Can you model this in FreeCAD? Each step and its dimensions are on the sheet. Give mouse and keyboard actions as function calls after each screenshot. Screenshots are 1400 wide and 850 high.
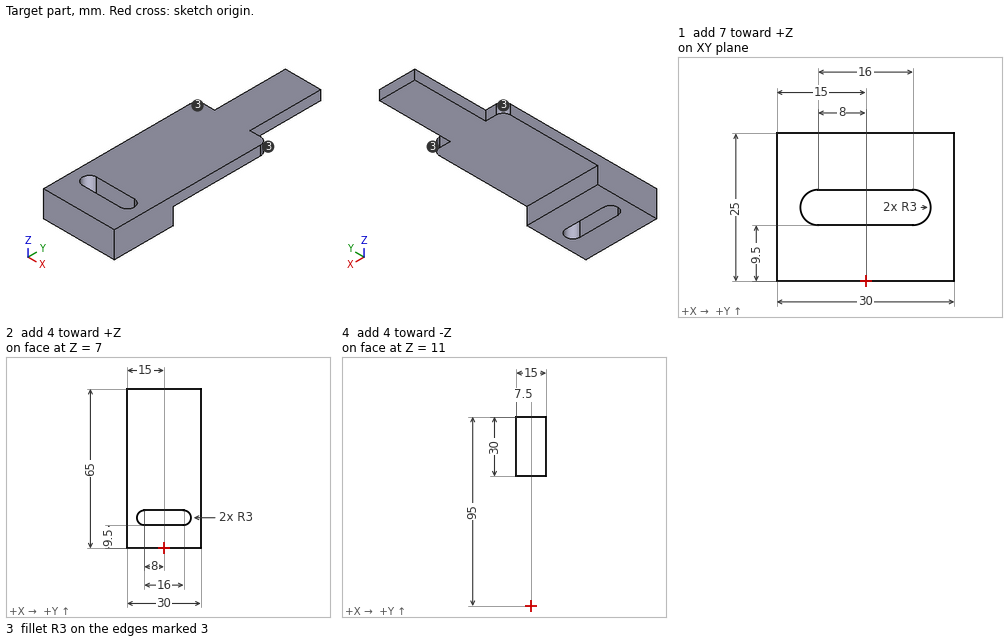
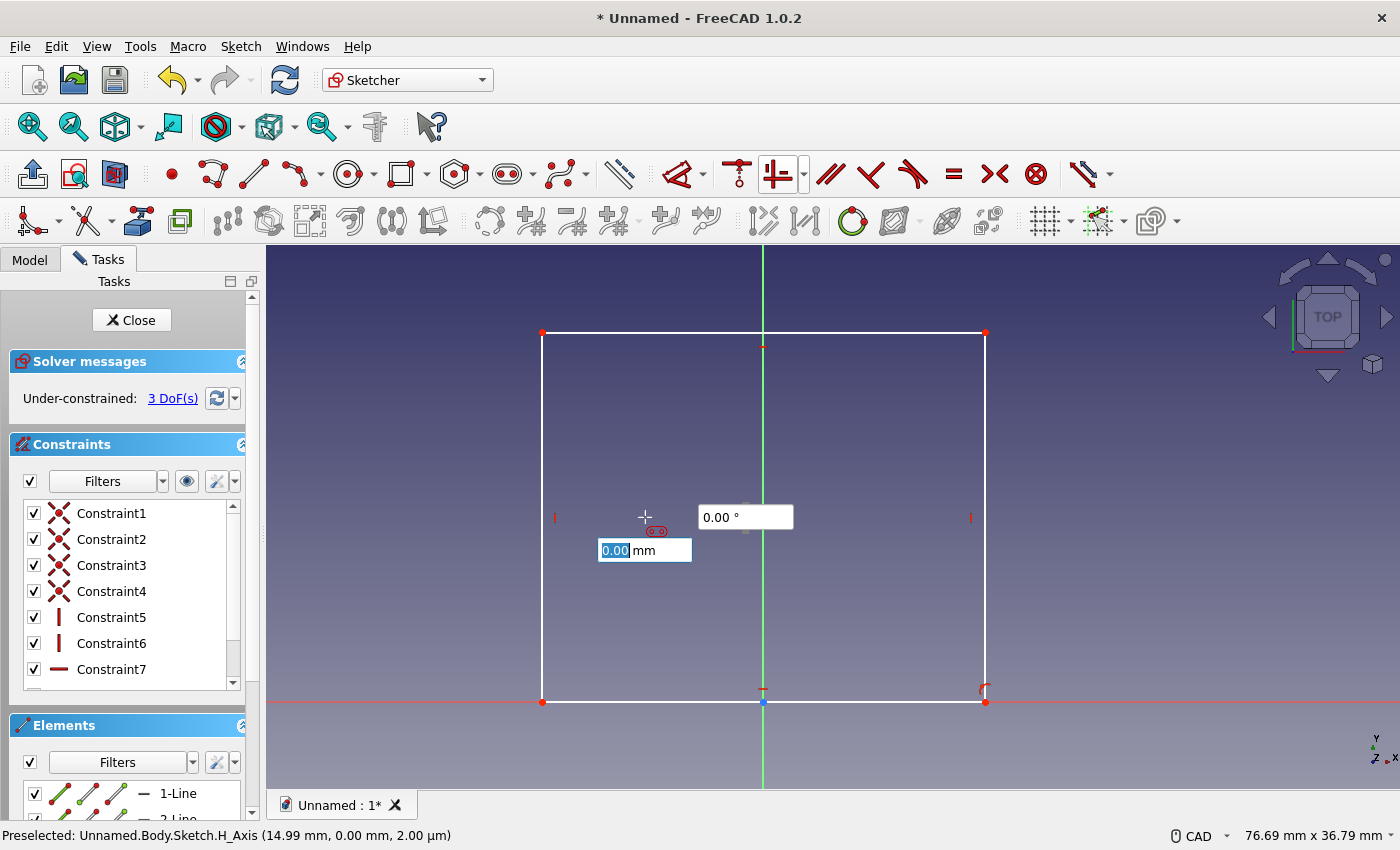
click(882, 517)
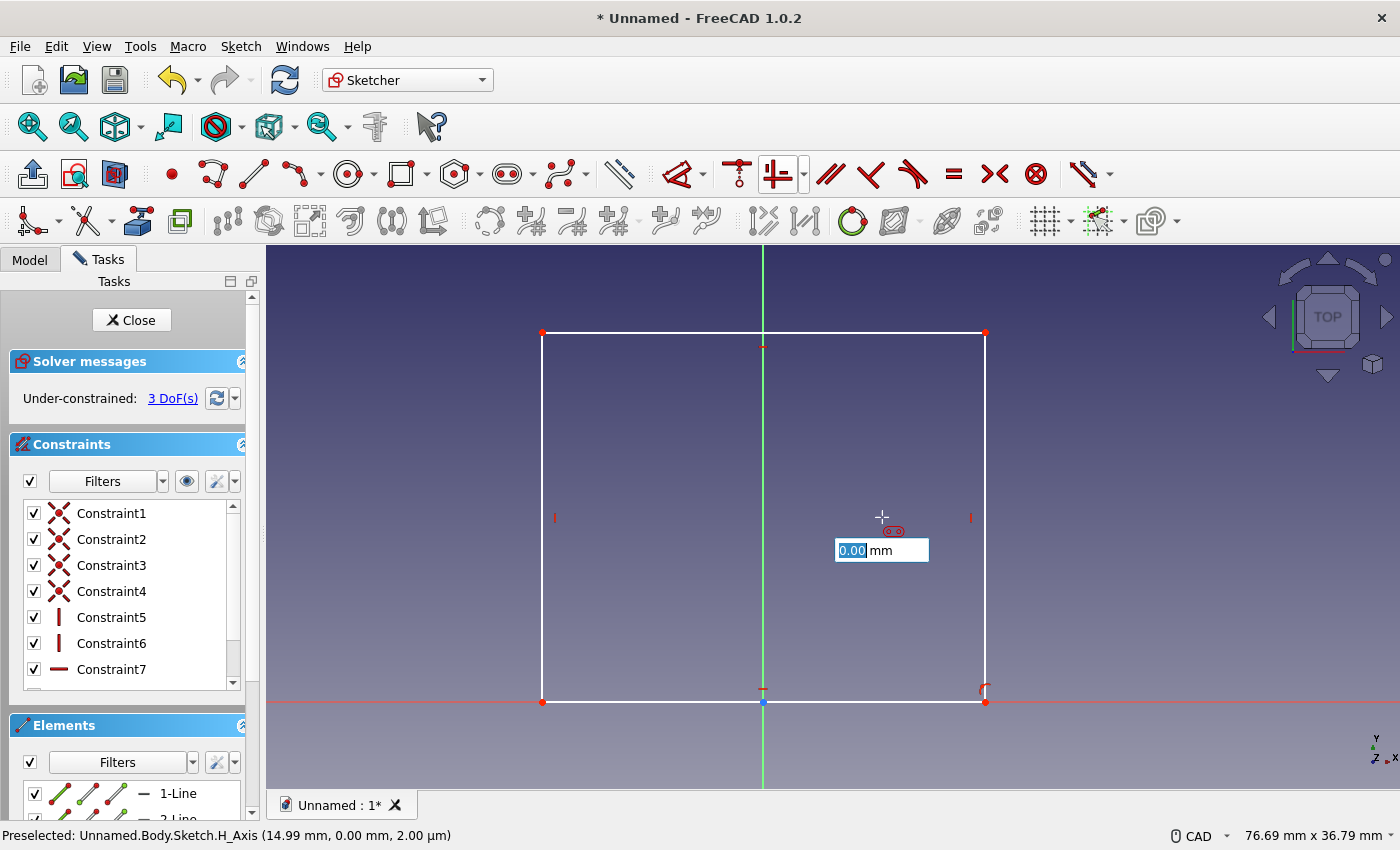
click(728, 473)
key(Escape)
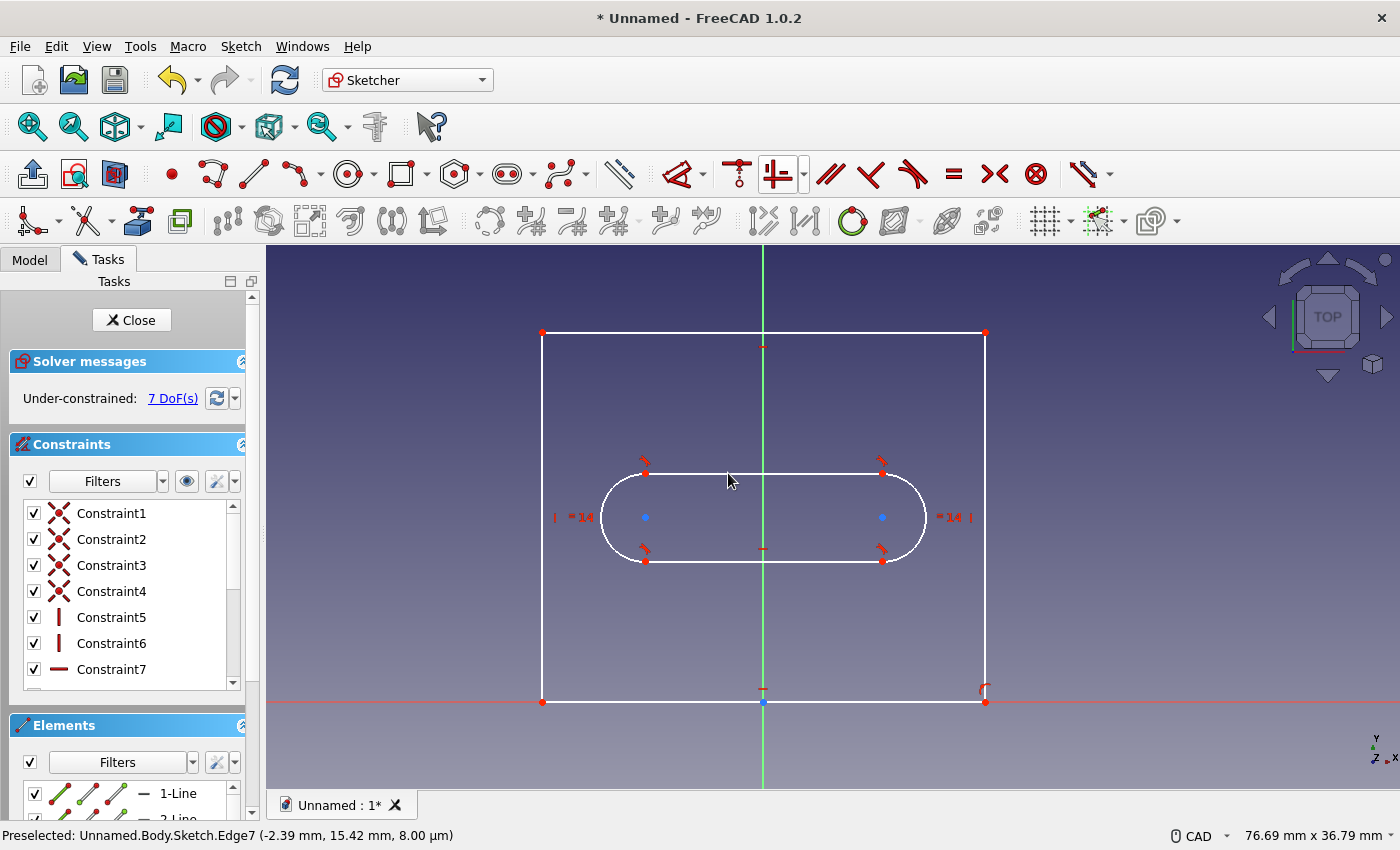
click(676, 174)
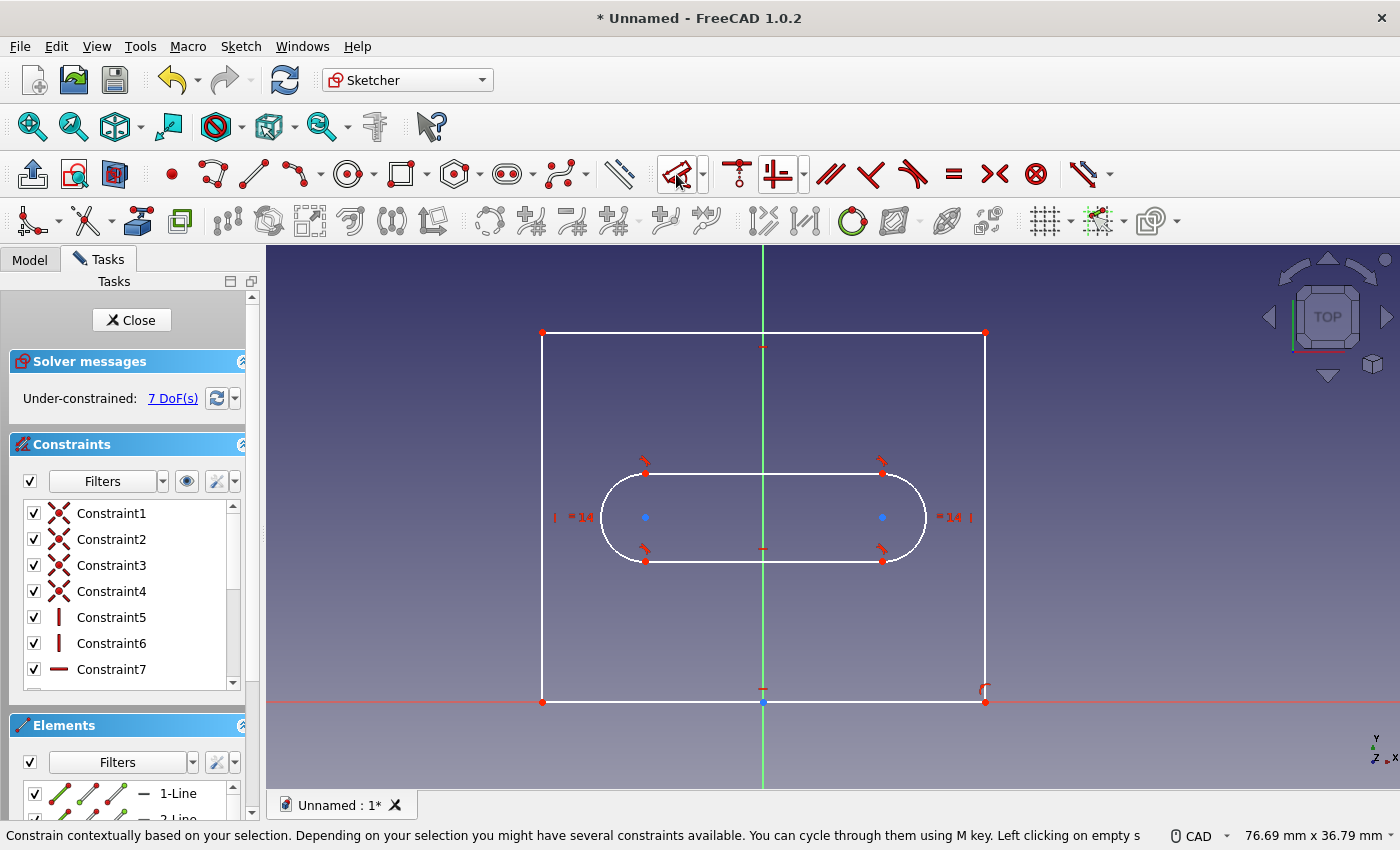
click(609, 492)
click(583, 473)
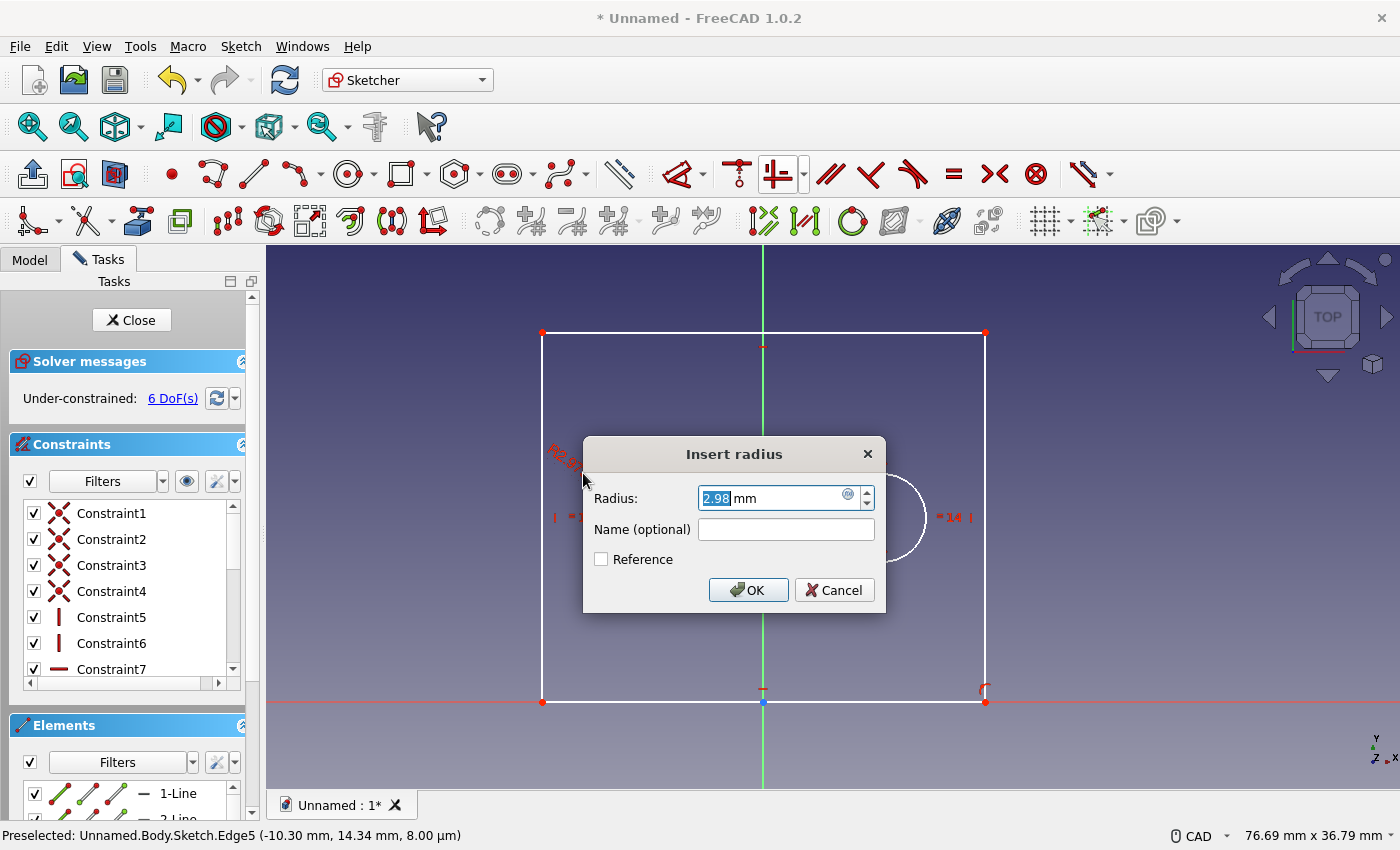
text(3)
key(Return)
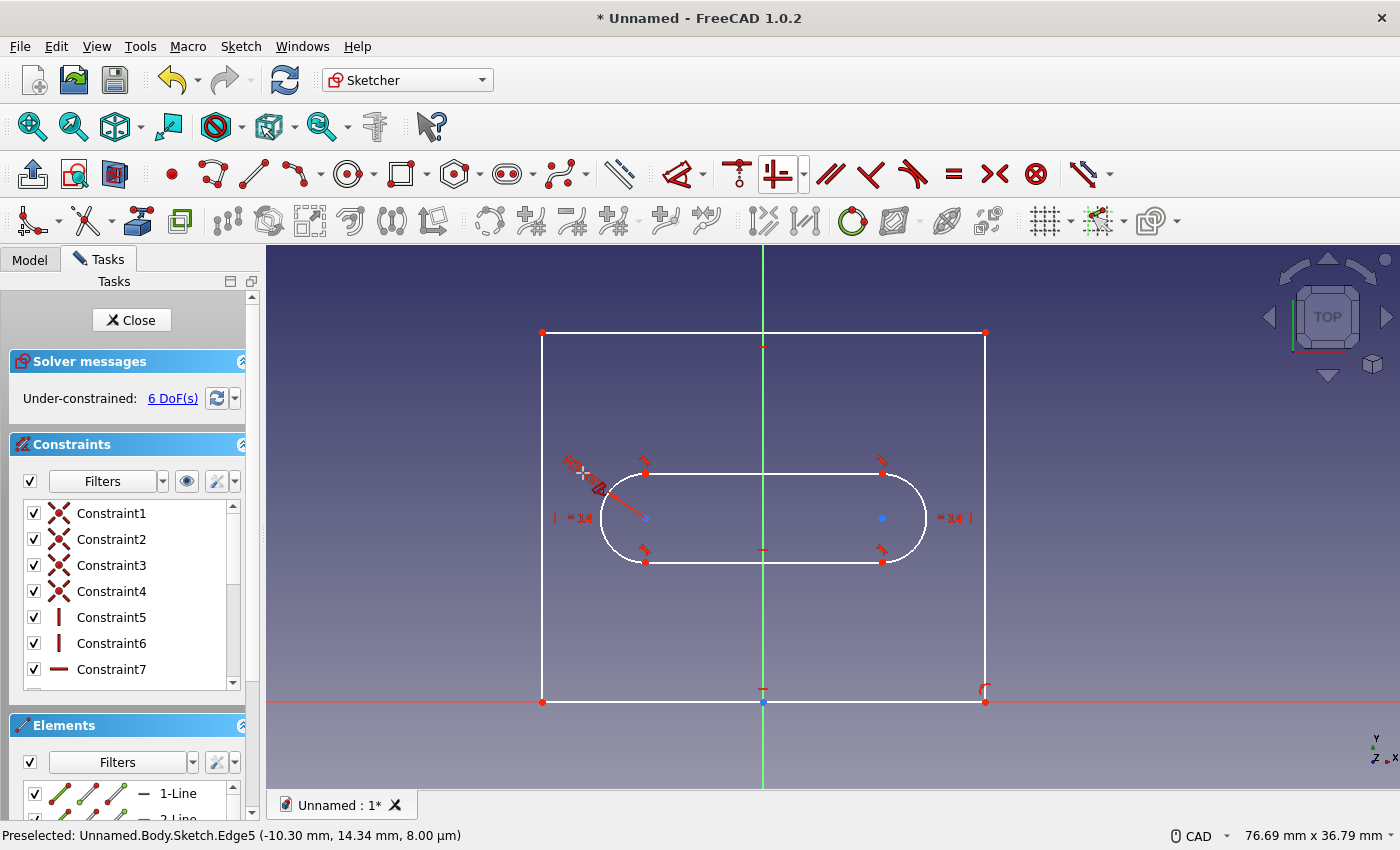
click(542, 444)
click(508, 518)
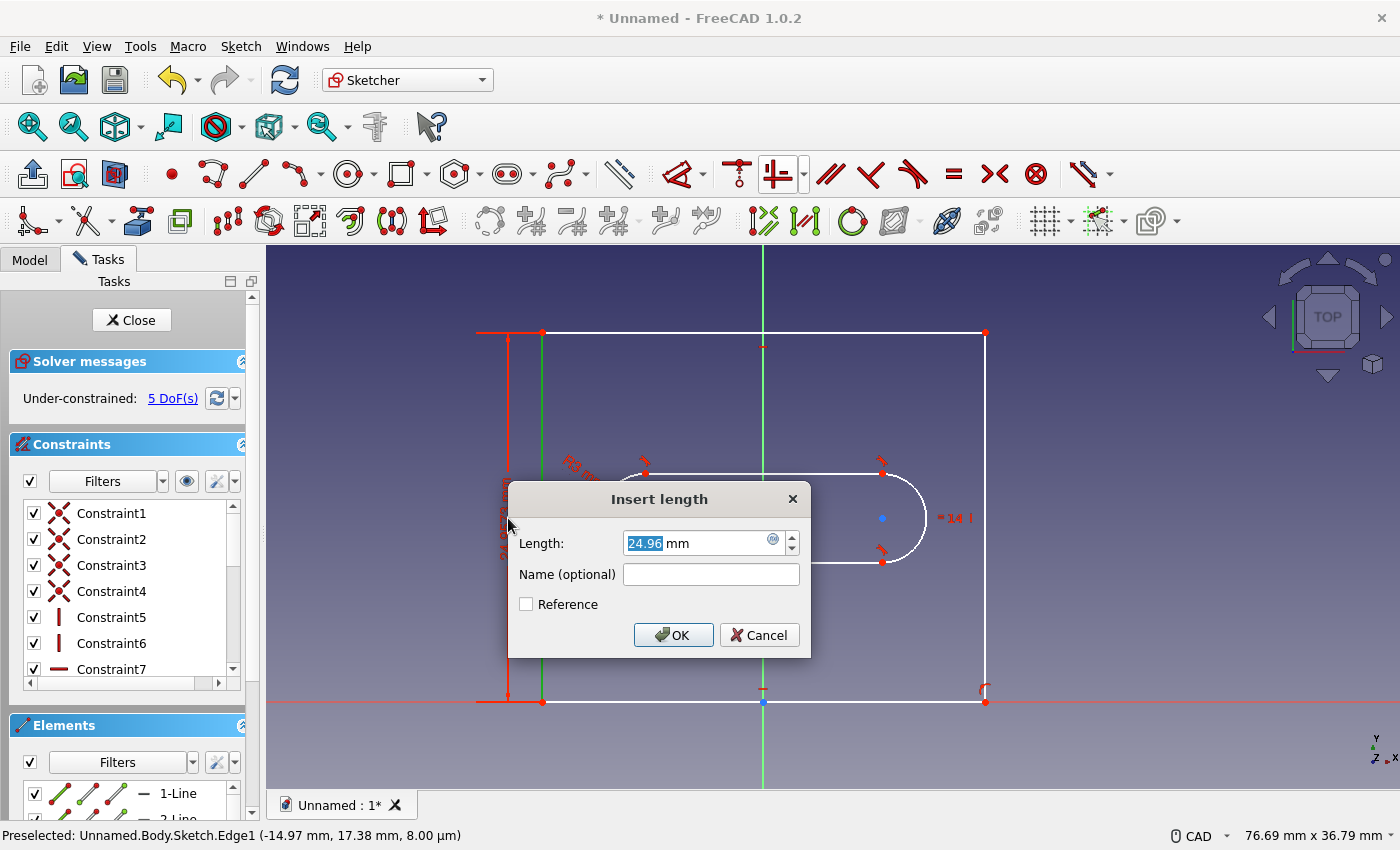
text(25)
key(Return)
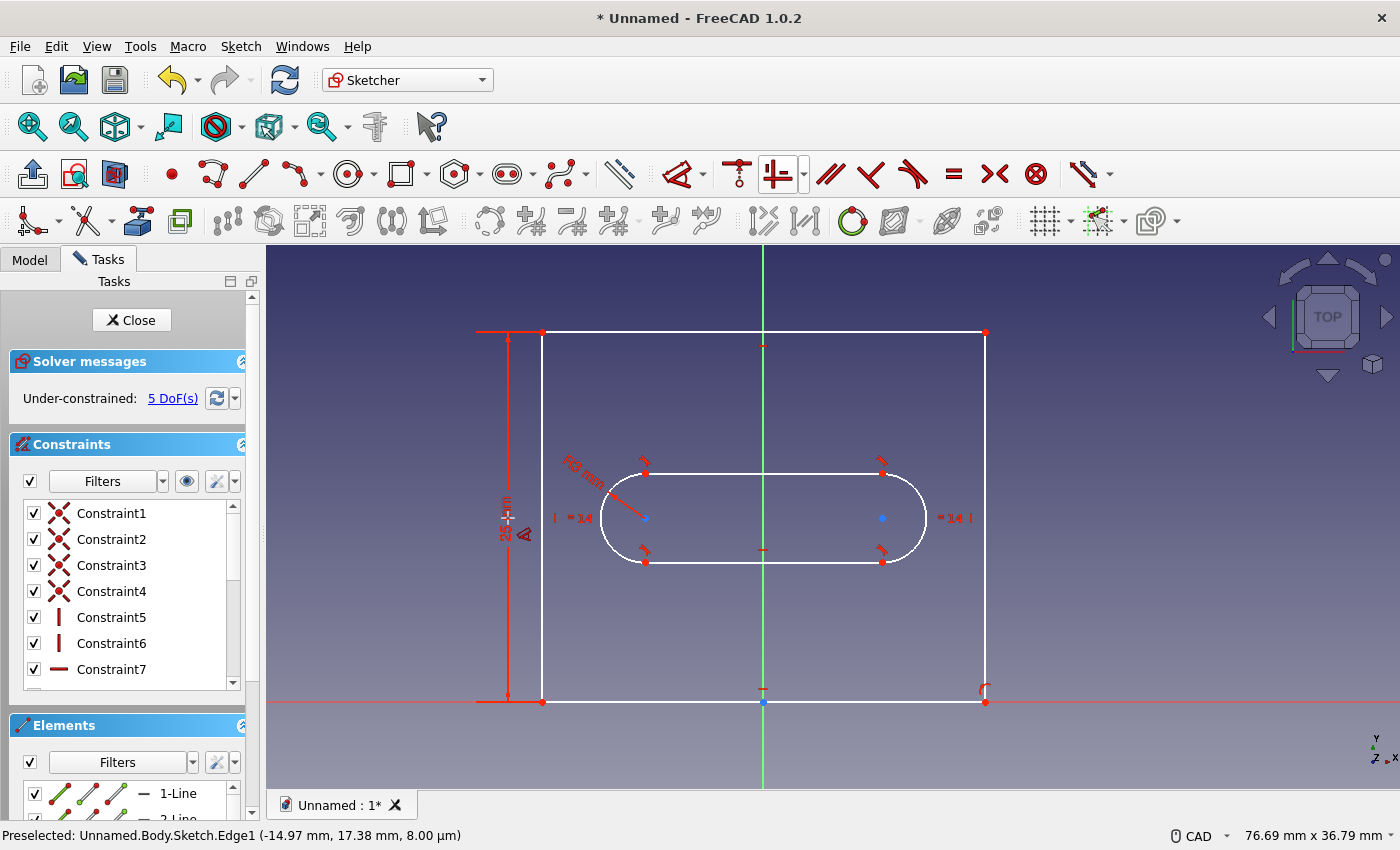
click(675, 702)
click(662, 736)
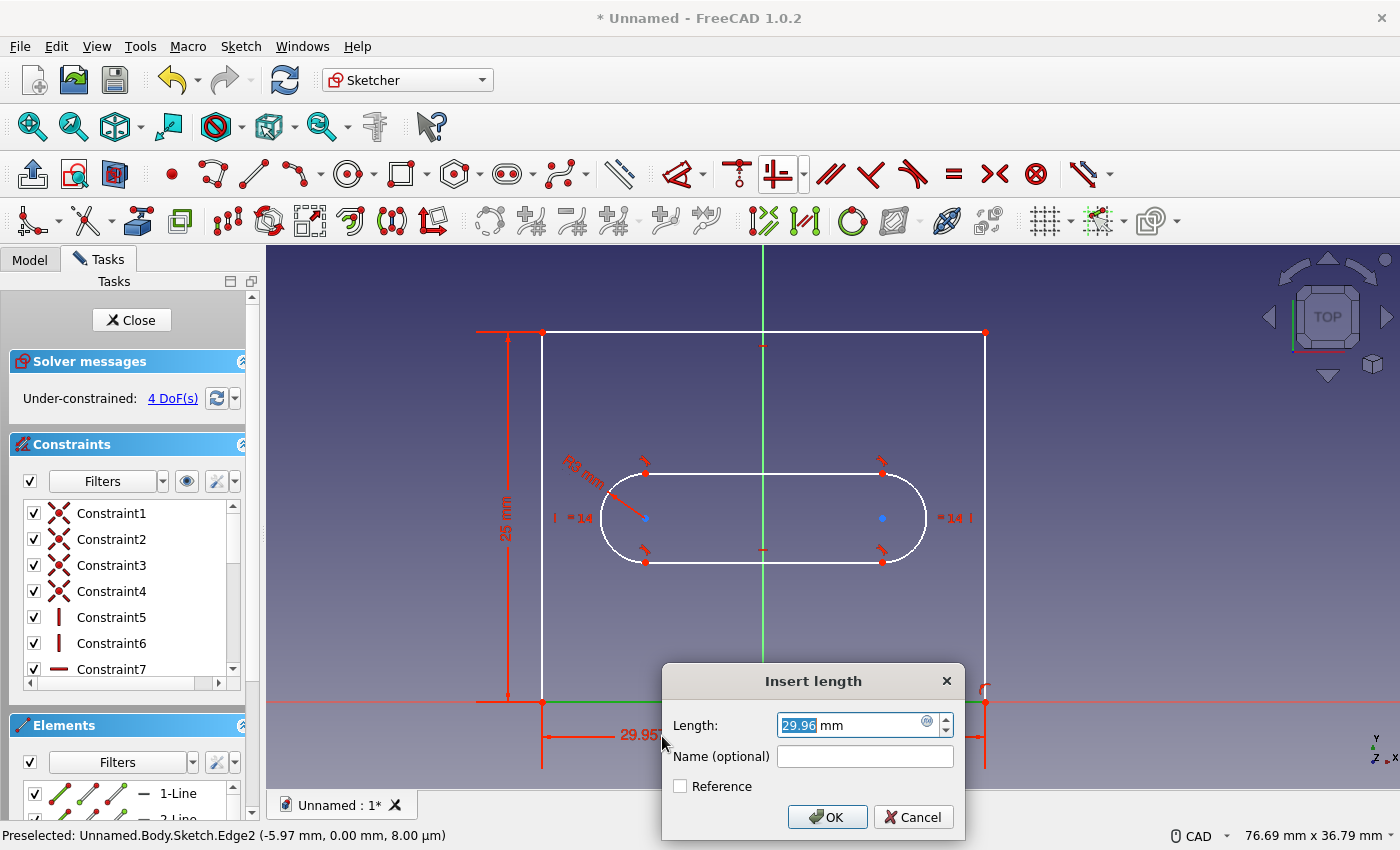
text(30)
key(Return)